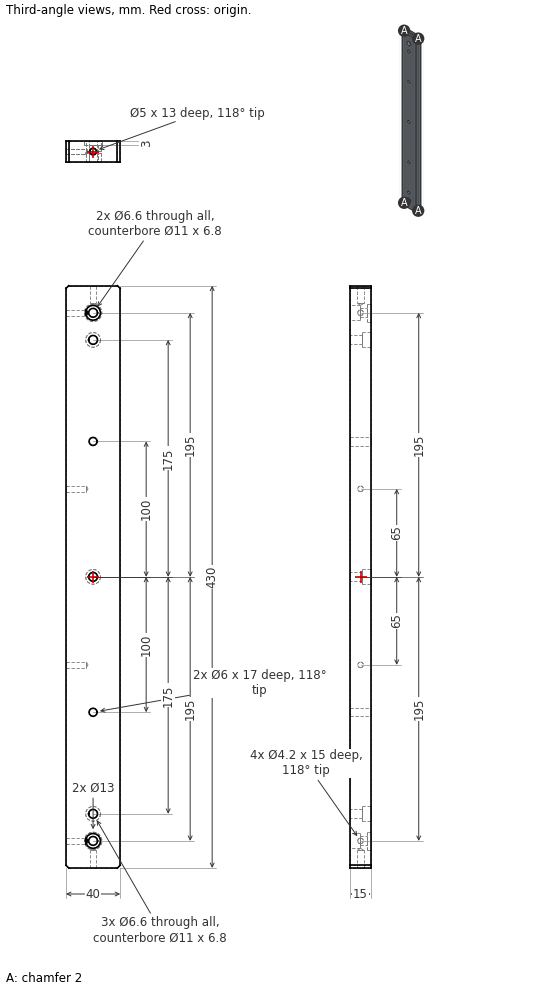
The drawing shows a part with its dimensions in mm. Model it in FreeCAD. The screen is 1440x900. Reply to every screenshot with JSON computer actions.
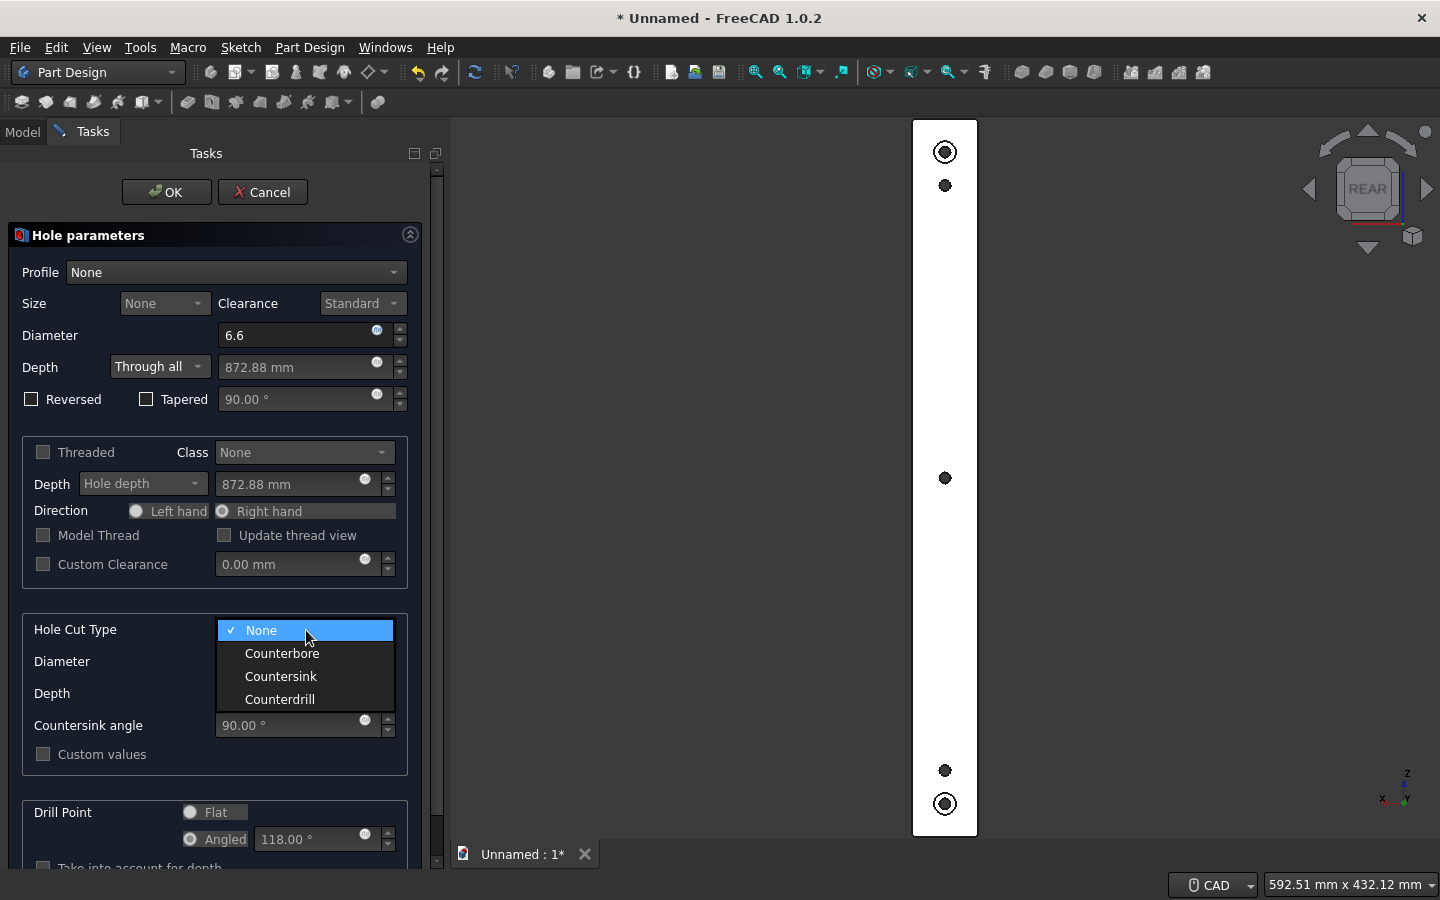
{"action": "left_click", "coordinate": [304, 654]}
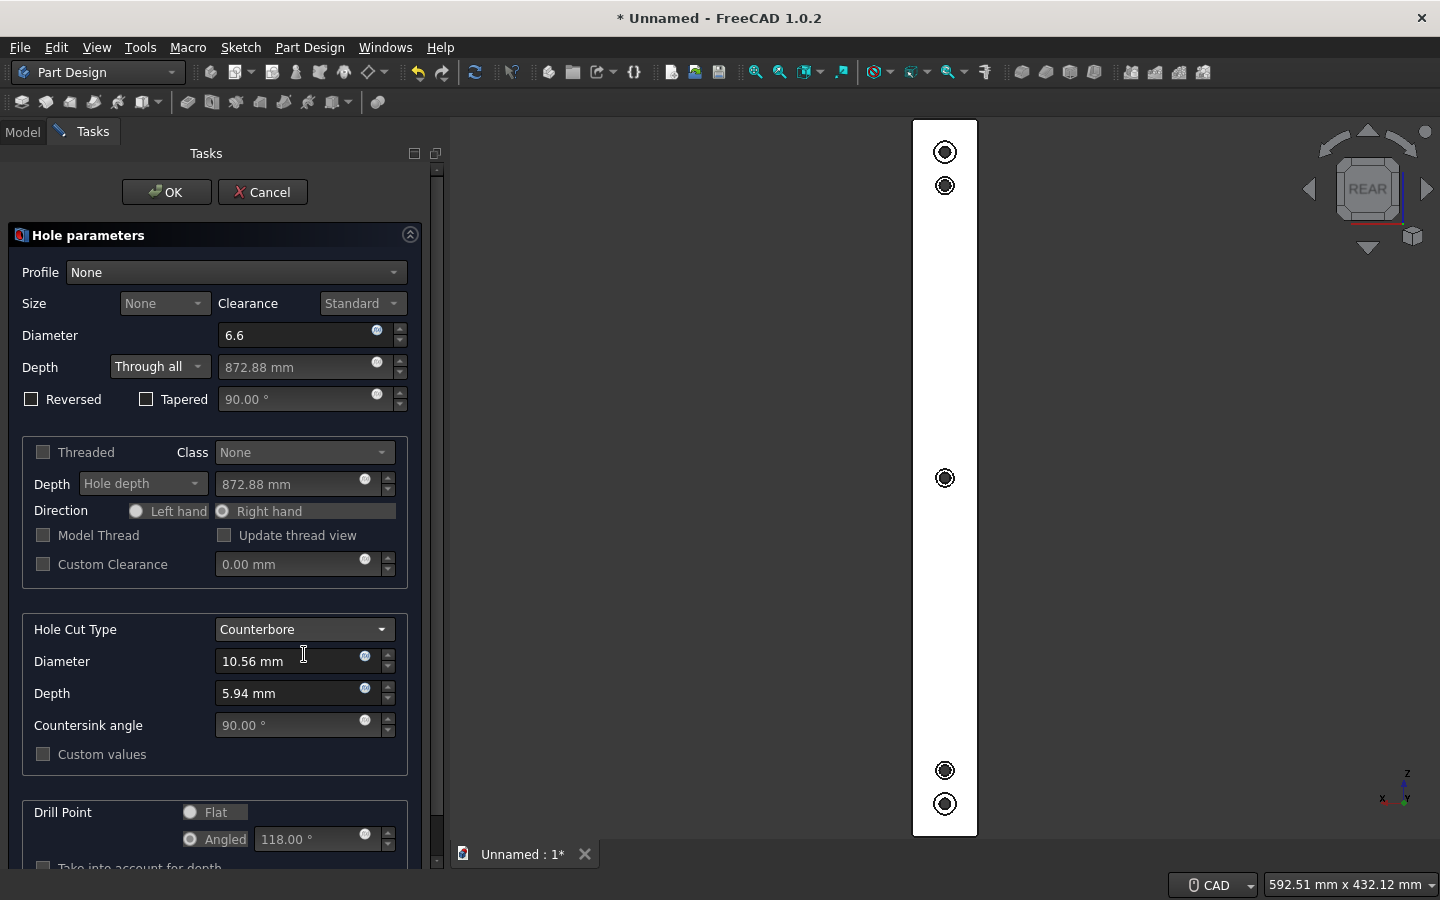
{"action": "triple_click", "coordinate": [298, 661]}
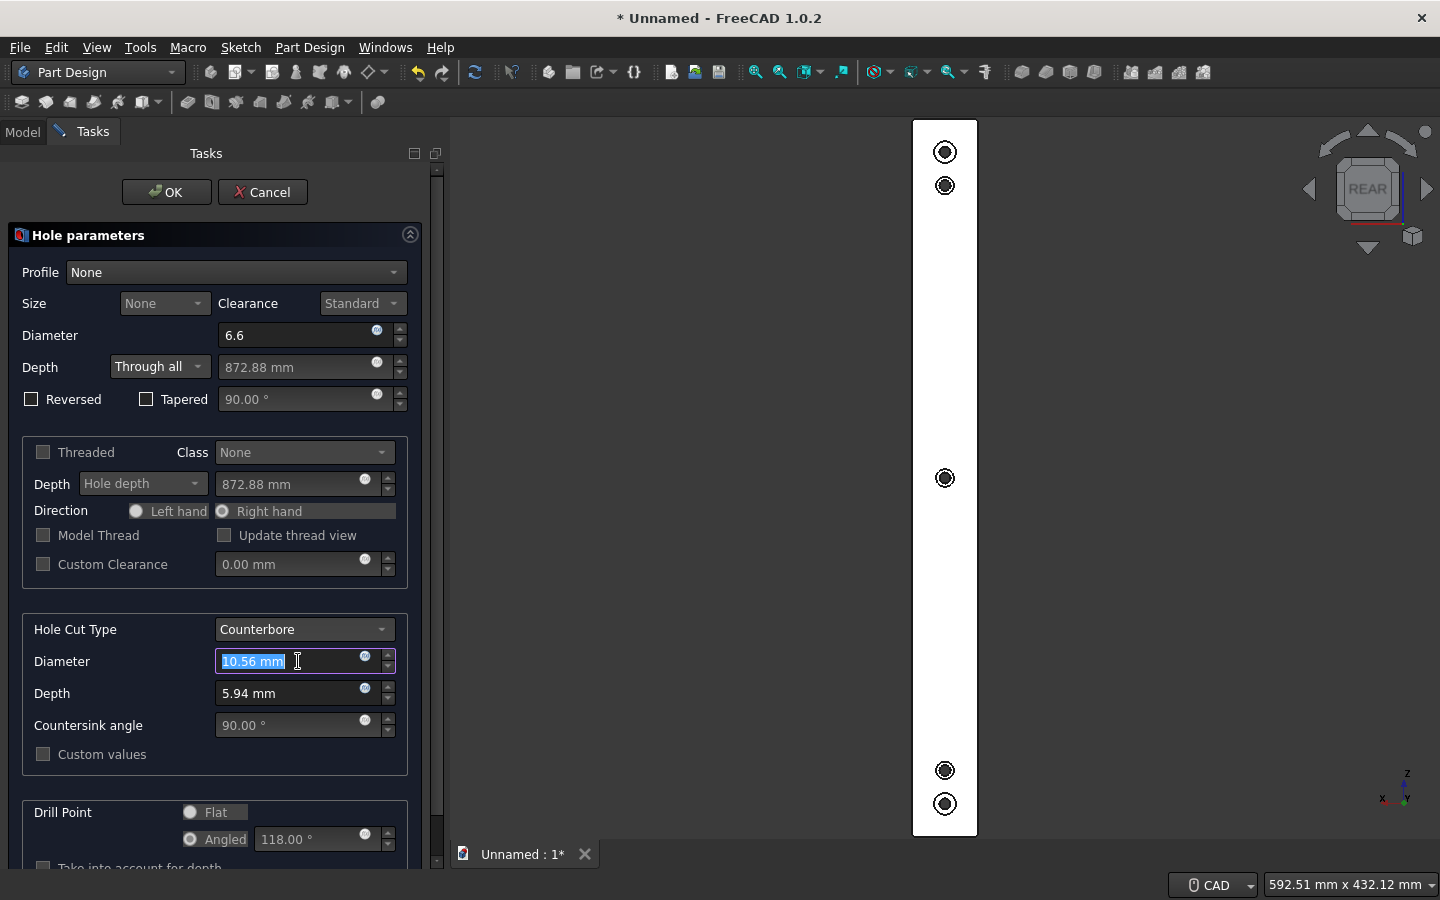
{"action": "type", "text": "11"}
{"action": "key", "text": "Tab"}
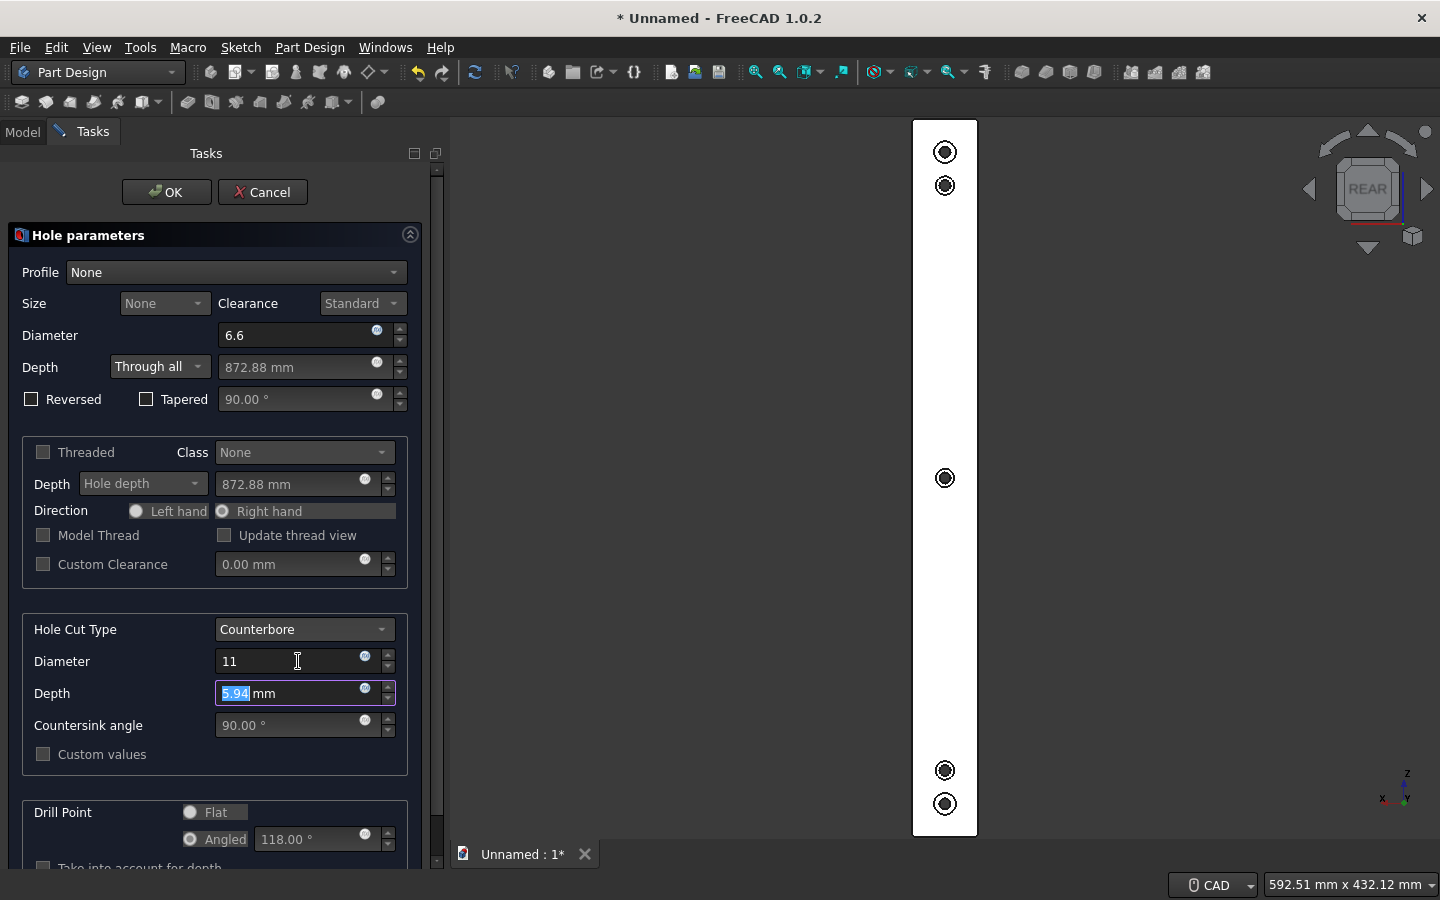
{"action": "type", "text": "6.8"}
{"action": "key", "text": "Tab"}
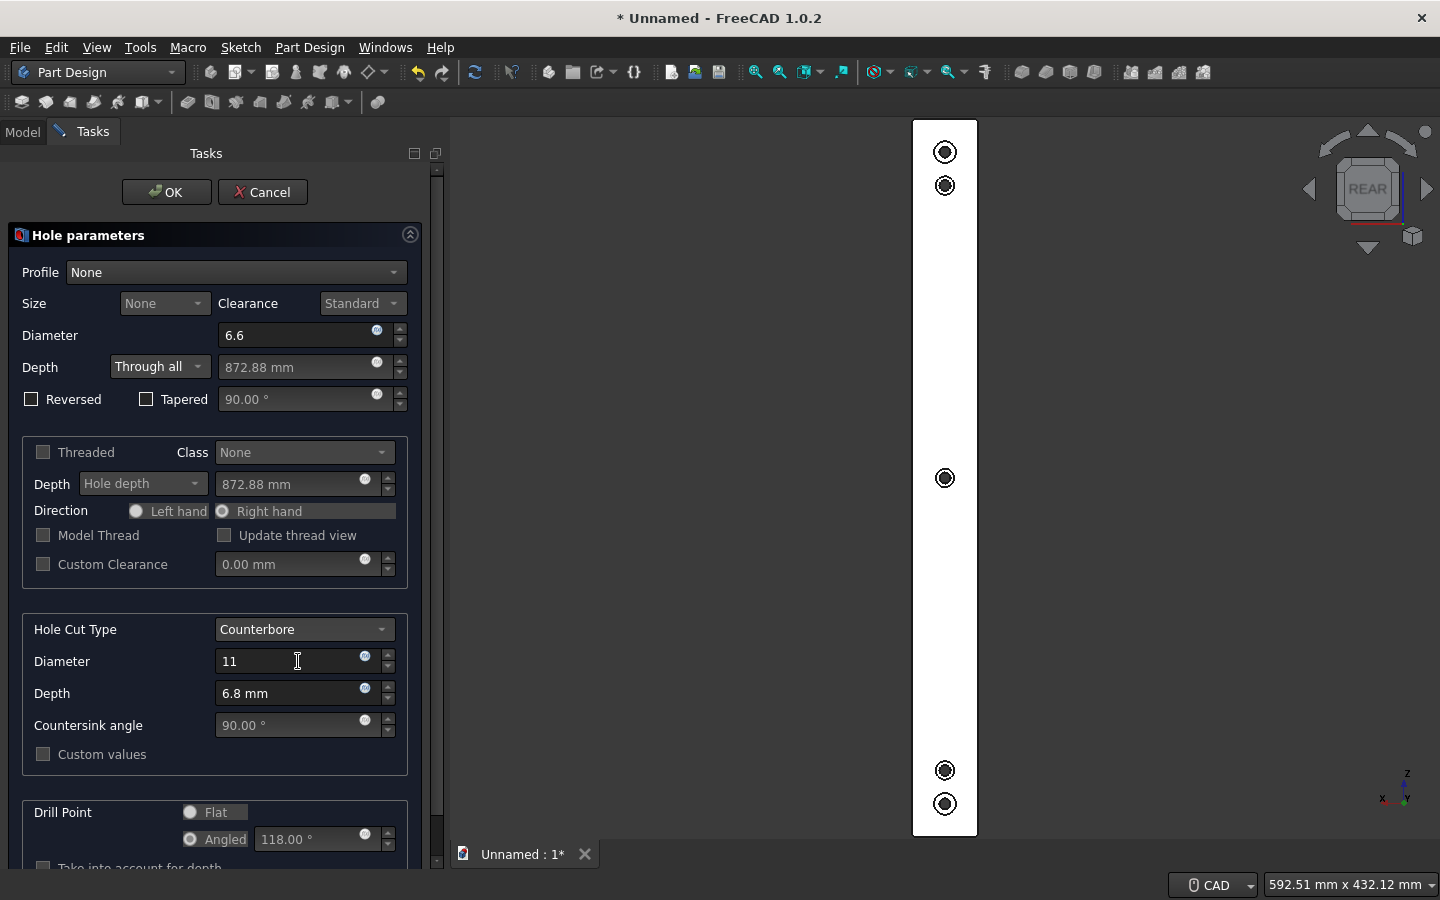
{"action": "left_click", "coordinate": [167, 192]}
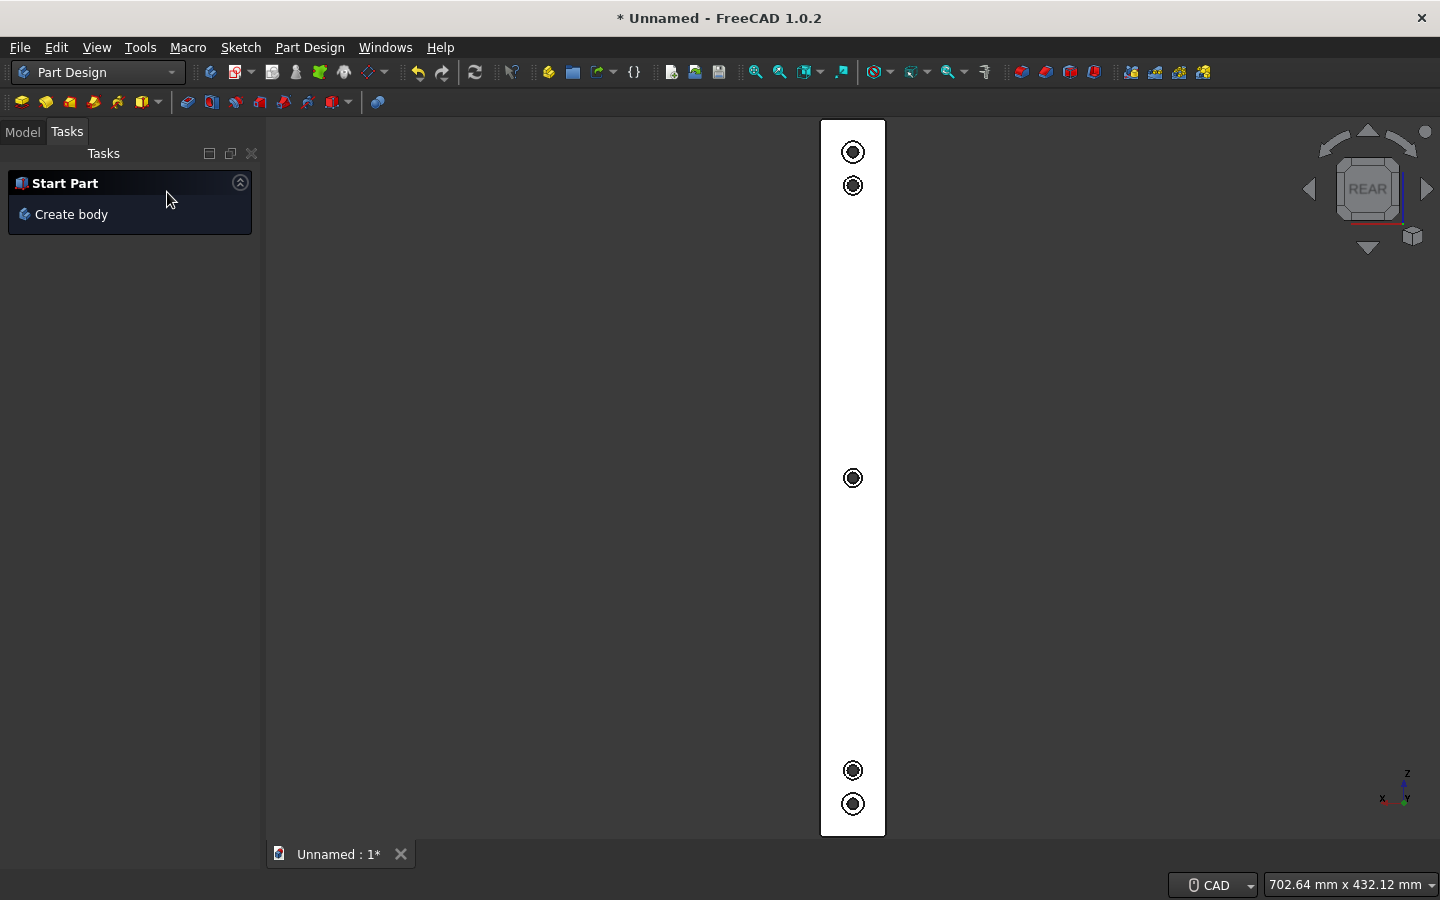
{"action": "key", "text": "0"}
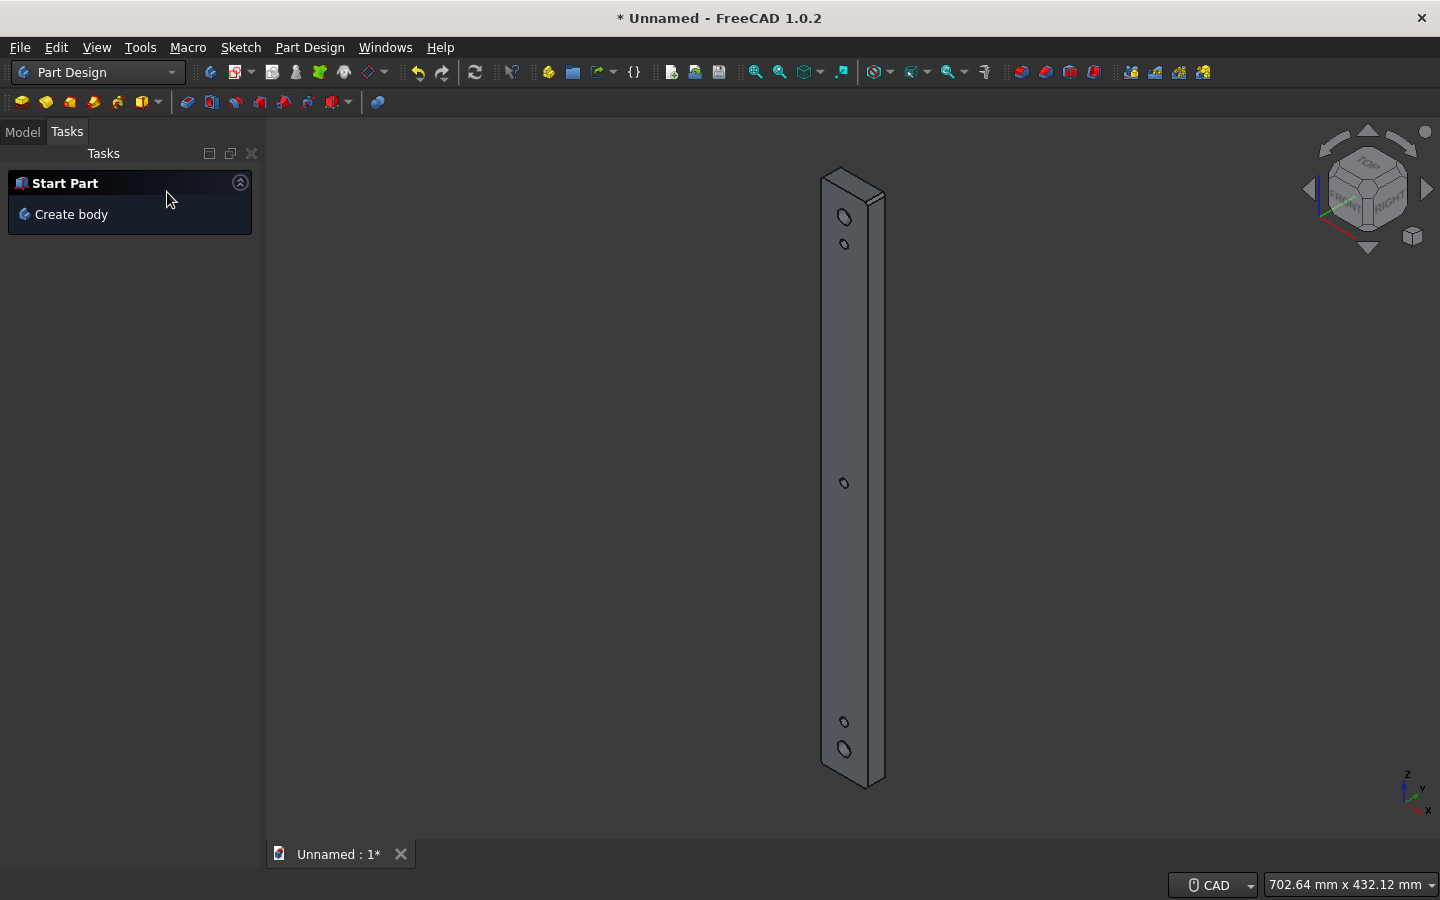
{"action": "left_click", "coordinate": [868, 189]}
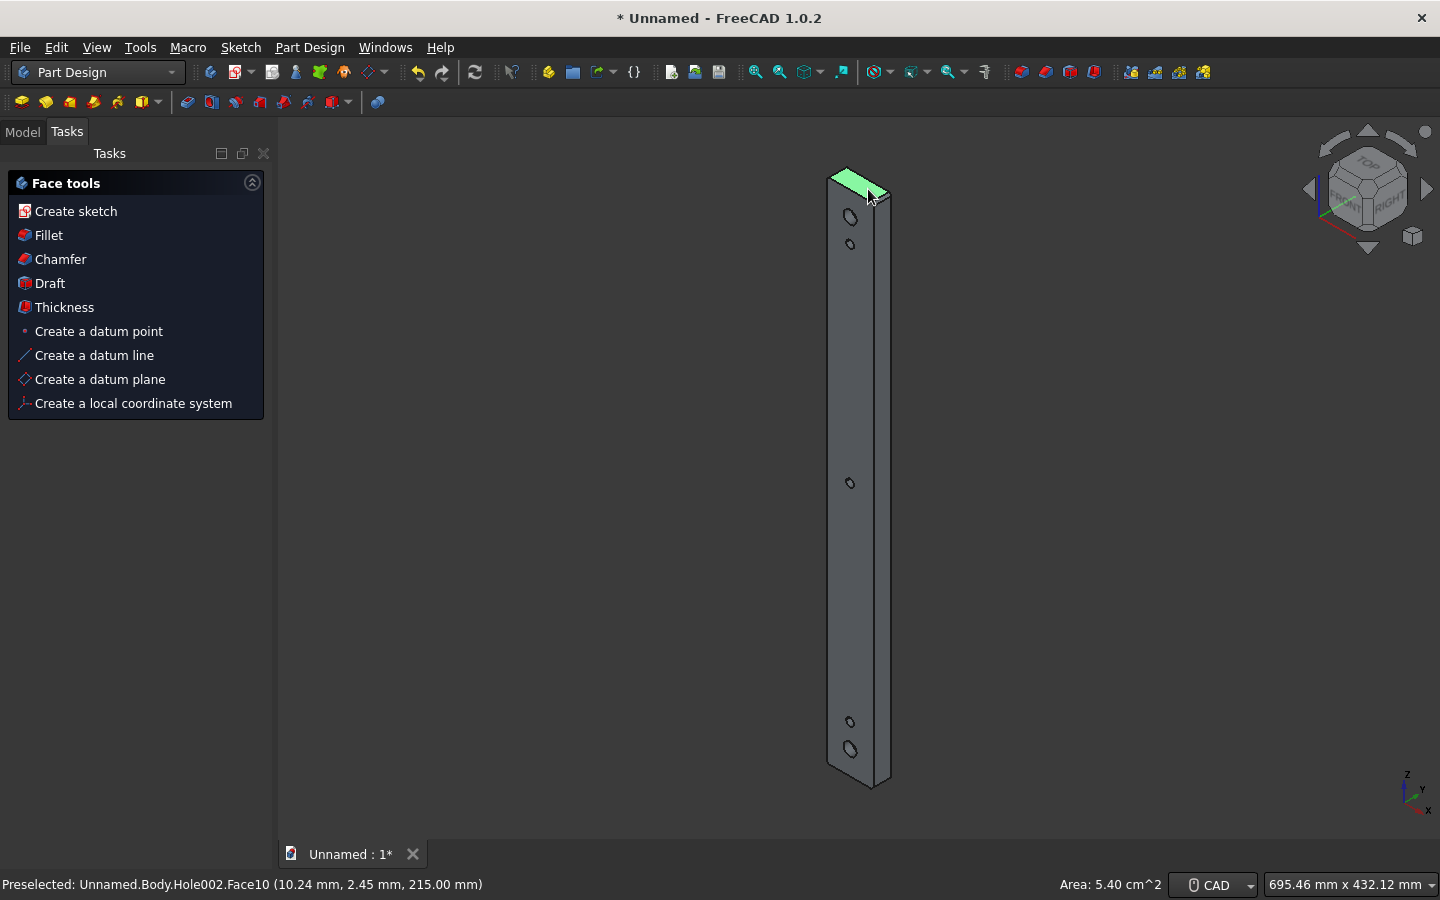
{"action": "left_click", "coordinate": [236, 72]}